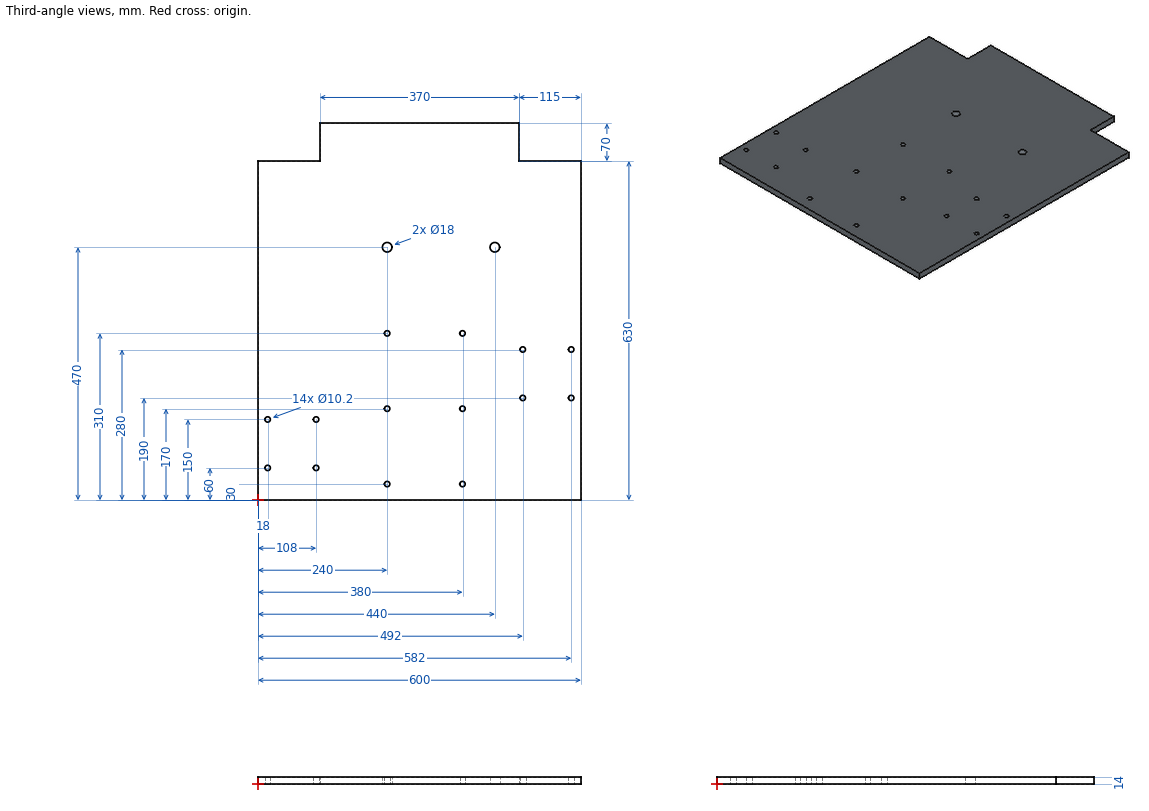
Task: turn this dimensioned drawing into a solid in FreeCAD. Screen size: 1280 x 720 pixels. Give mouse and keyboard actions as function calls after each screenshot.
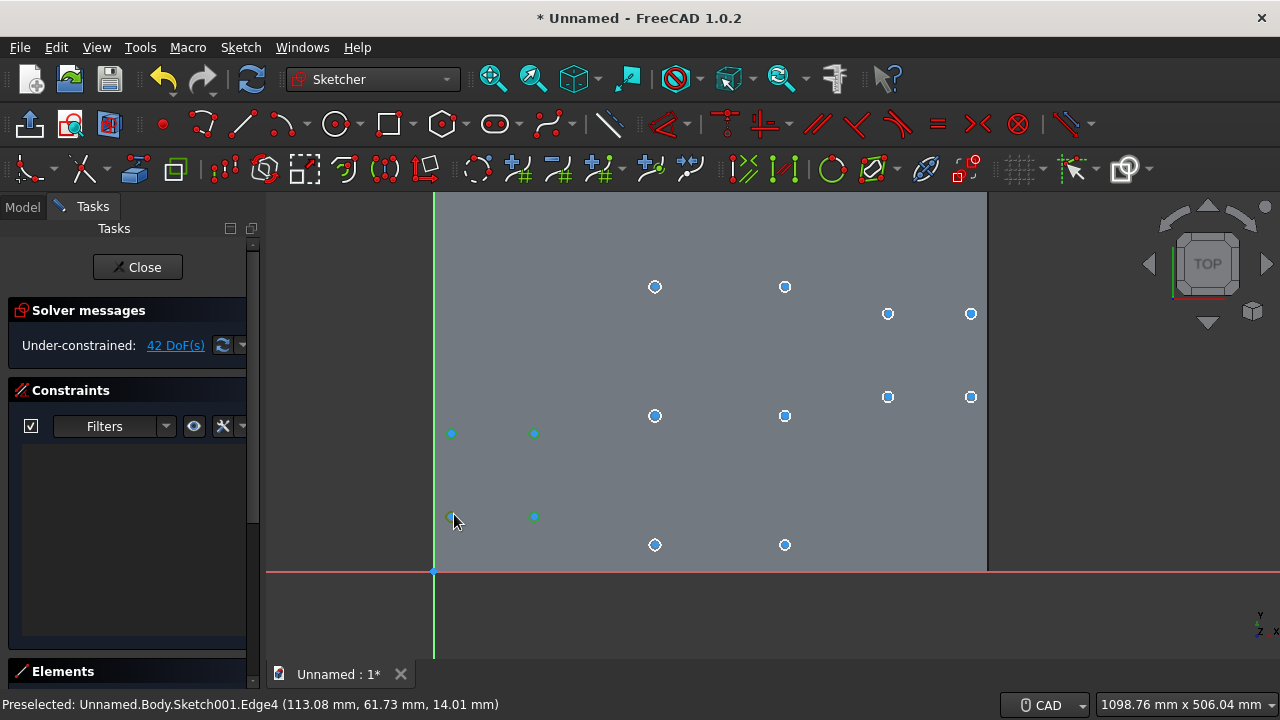
scroll(892, 310, up, 5)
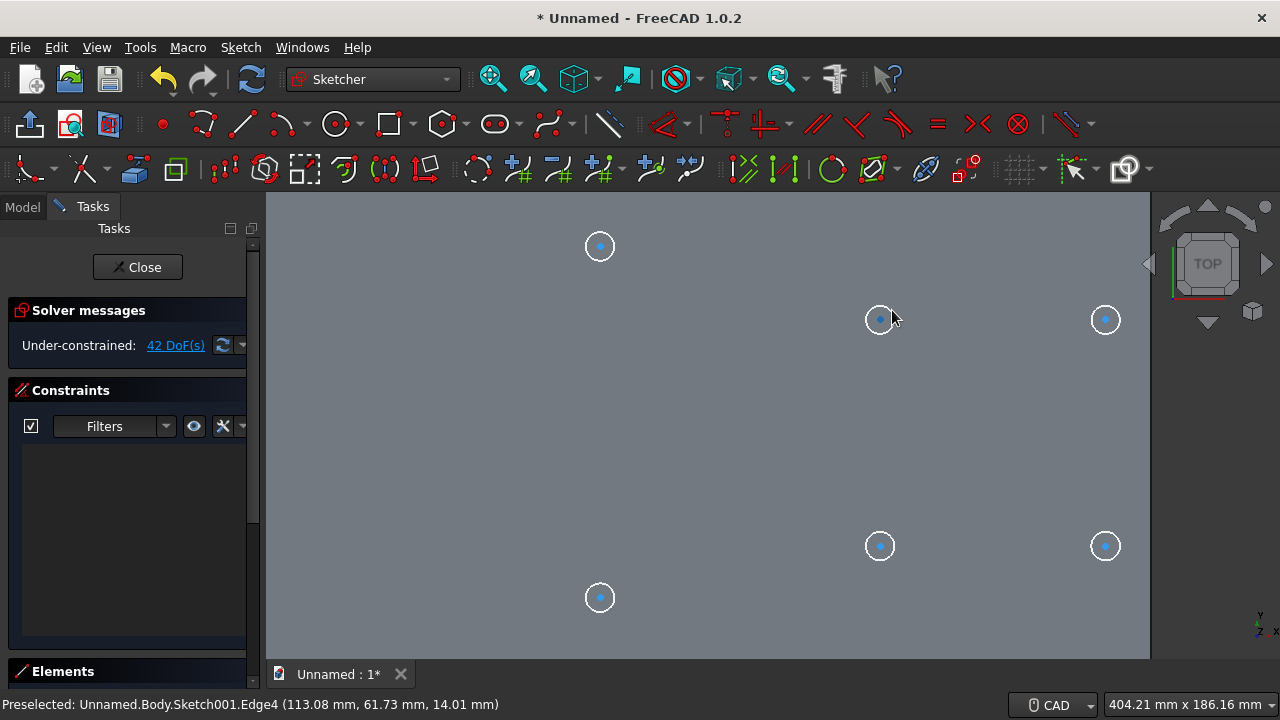
click(890, 310)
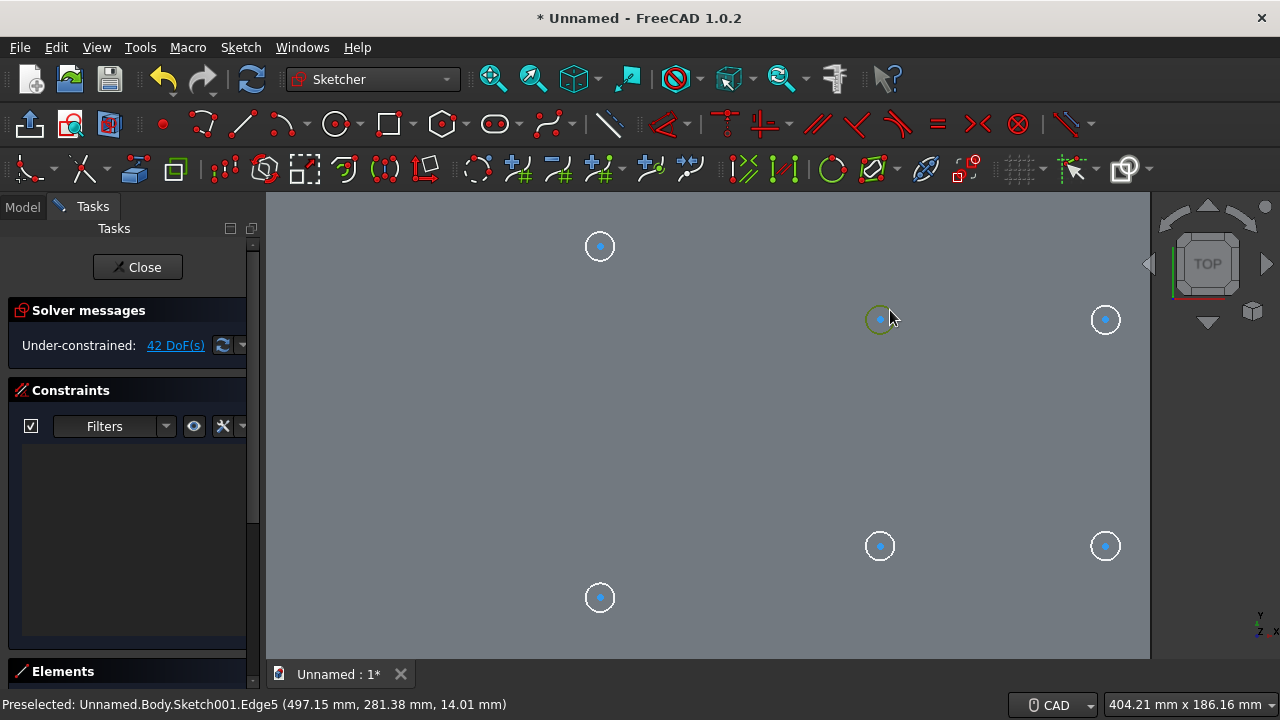
click(1096, 310)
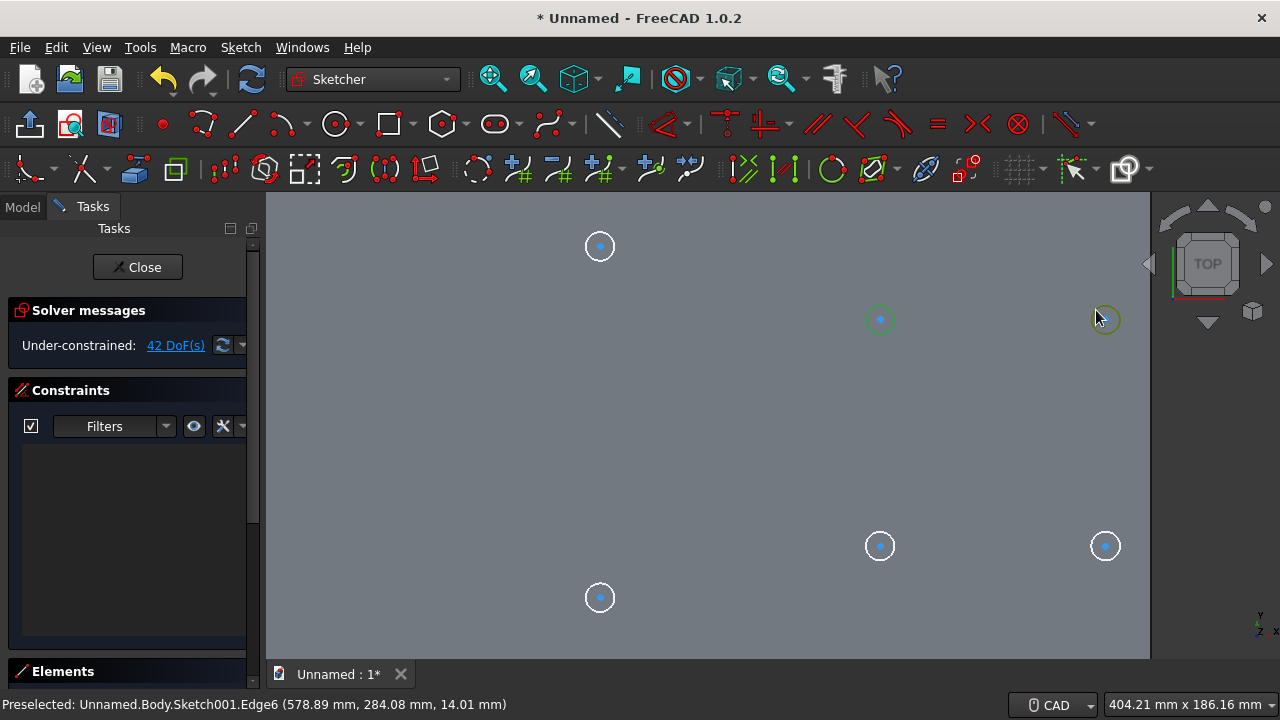
click(890, 536)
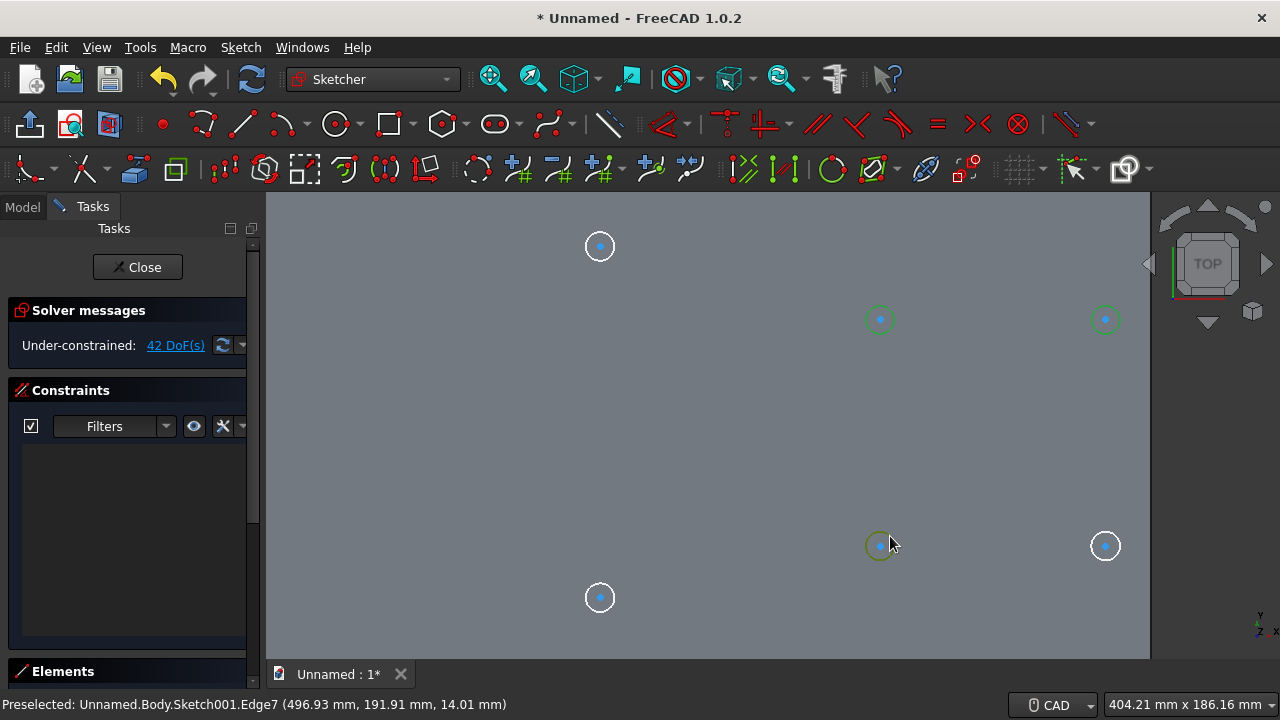
click(1096, 536)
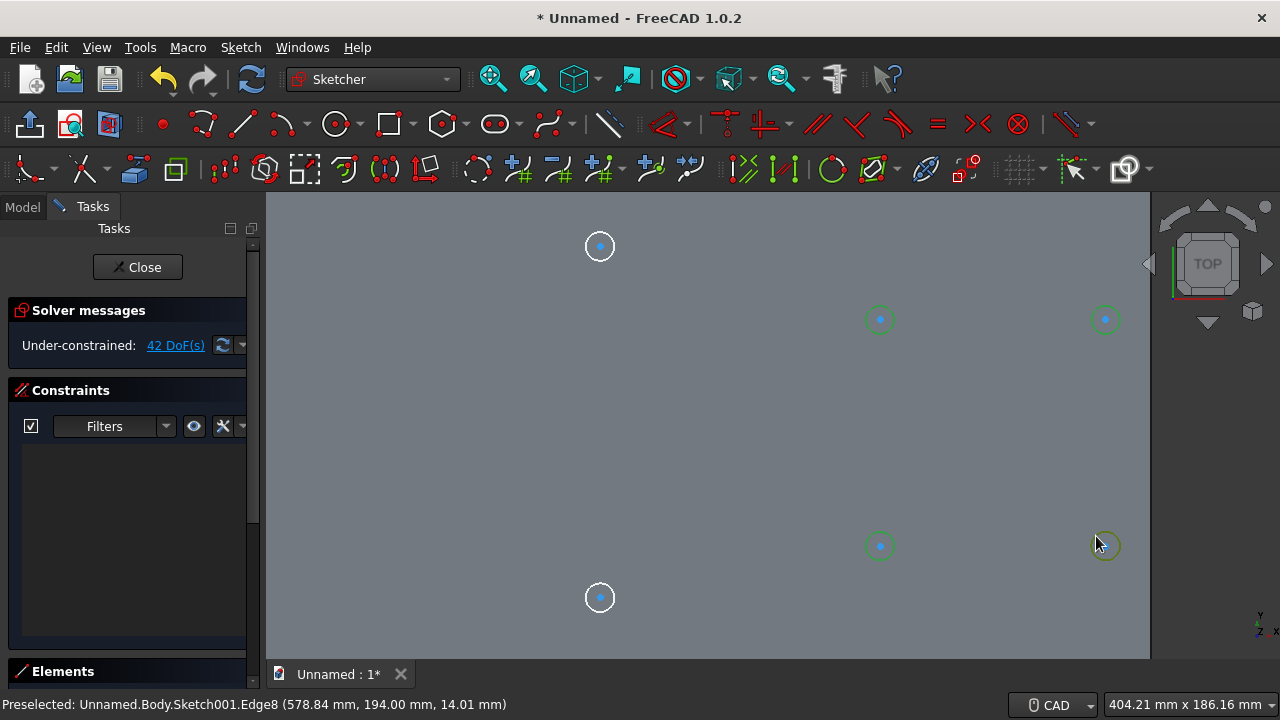
scroll(892, 309, down, 5)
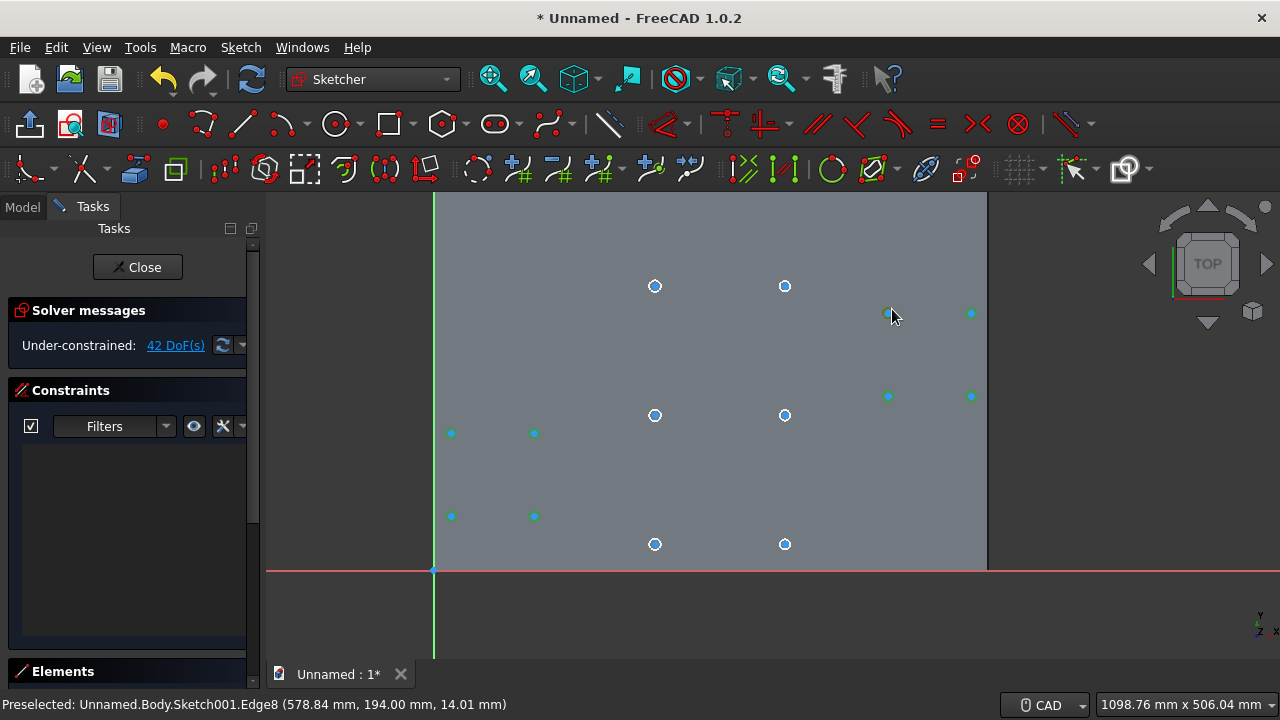
scroll(659, 282, up, 5)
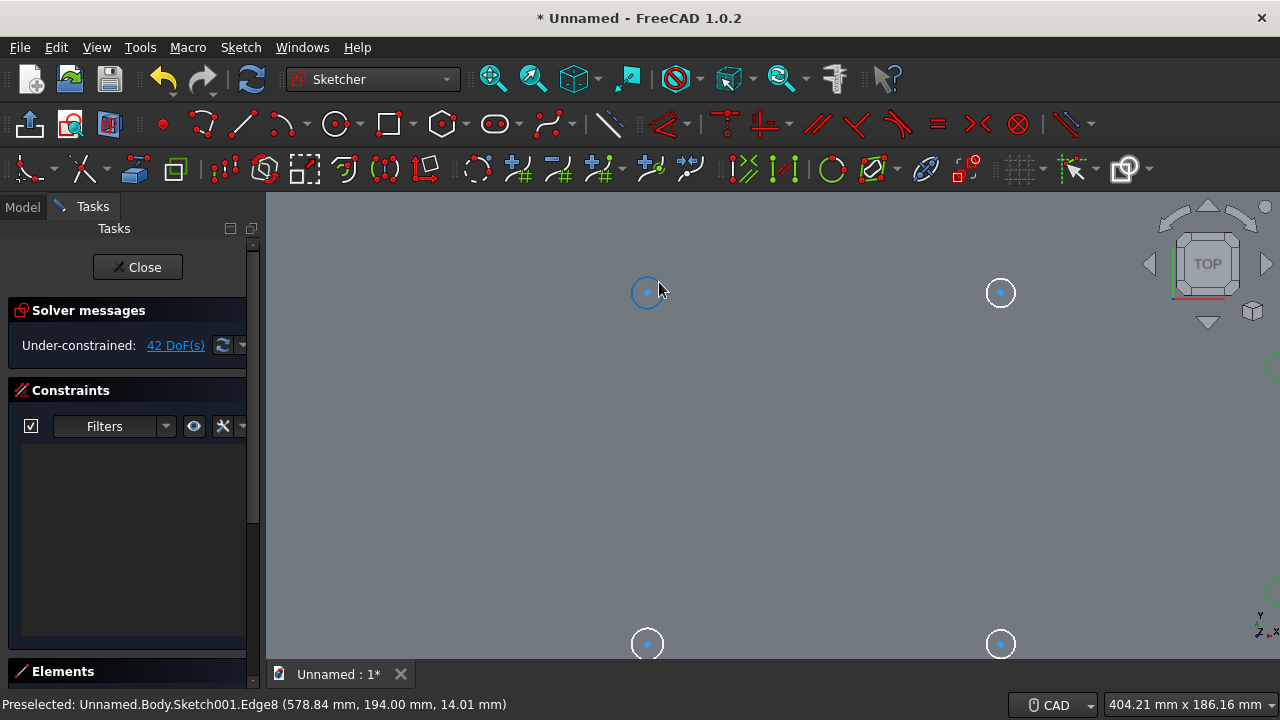
click(659, 282)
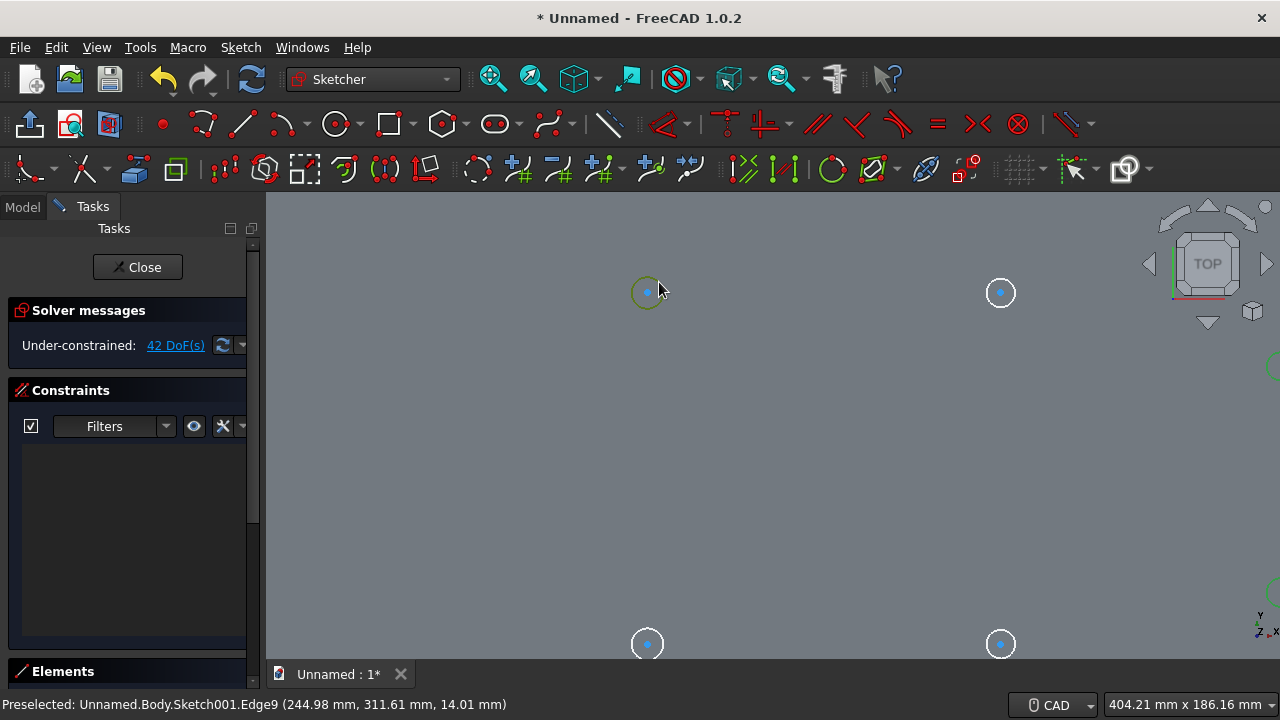
click(1011, 283)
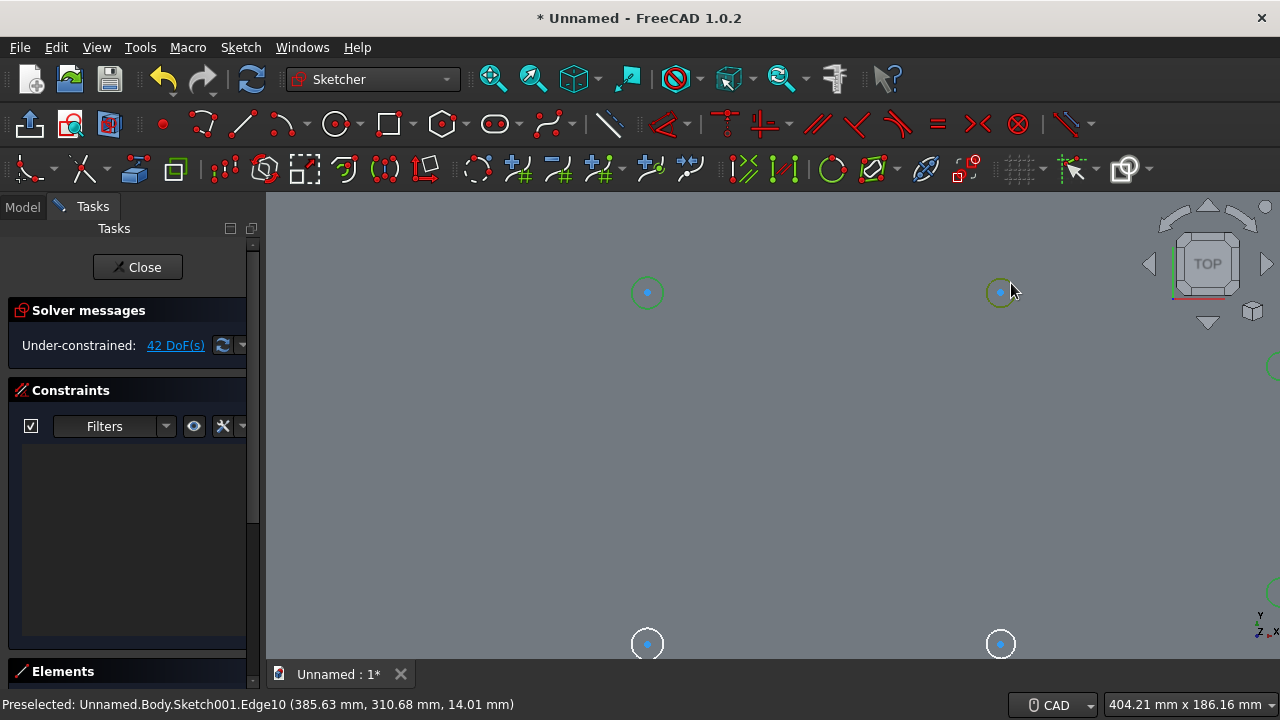
click(648, 628)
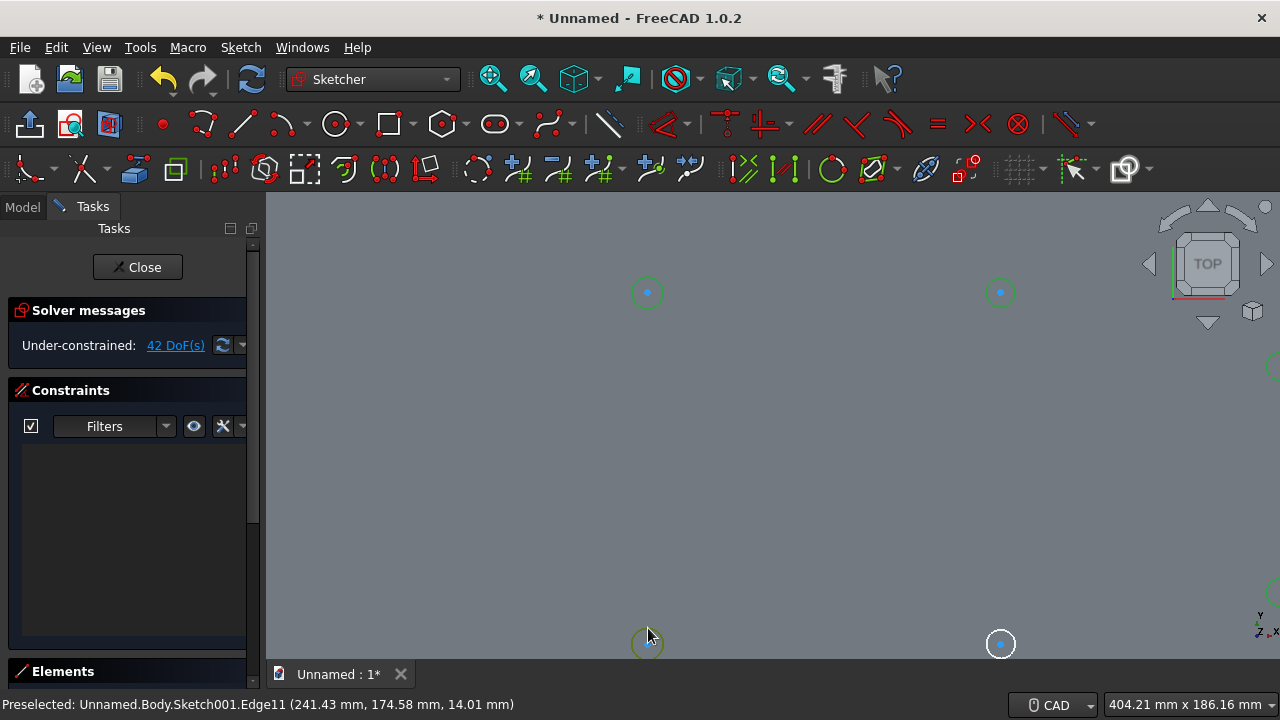
click(1001, 630)